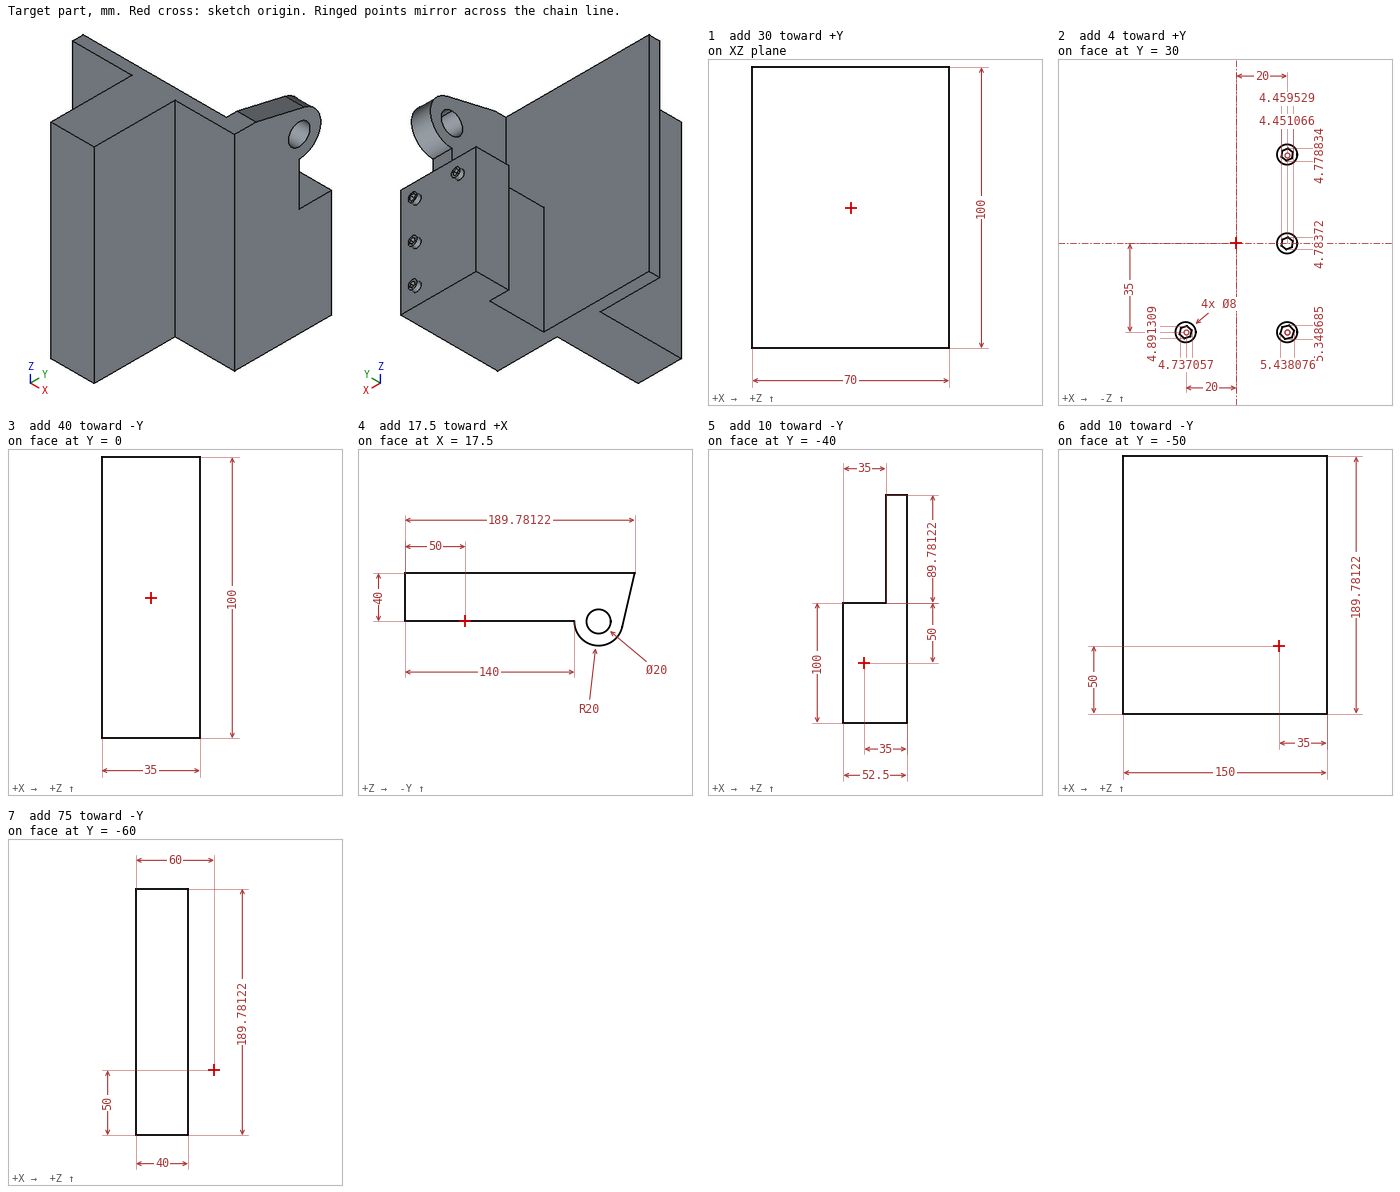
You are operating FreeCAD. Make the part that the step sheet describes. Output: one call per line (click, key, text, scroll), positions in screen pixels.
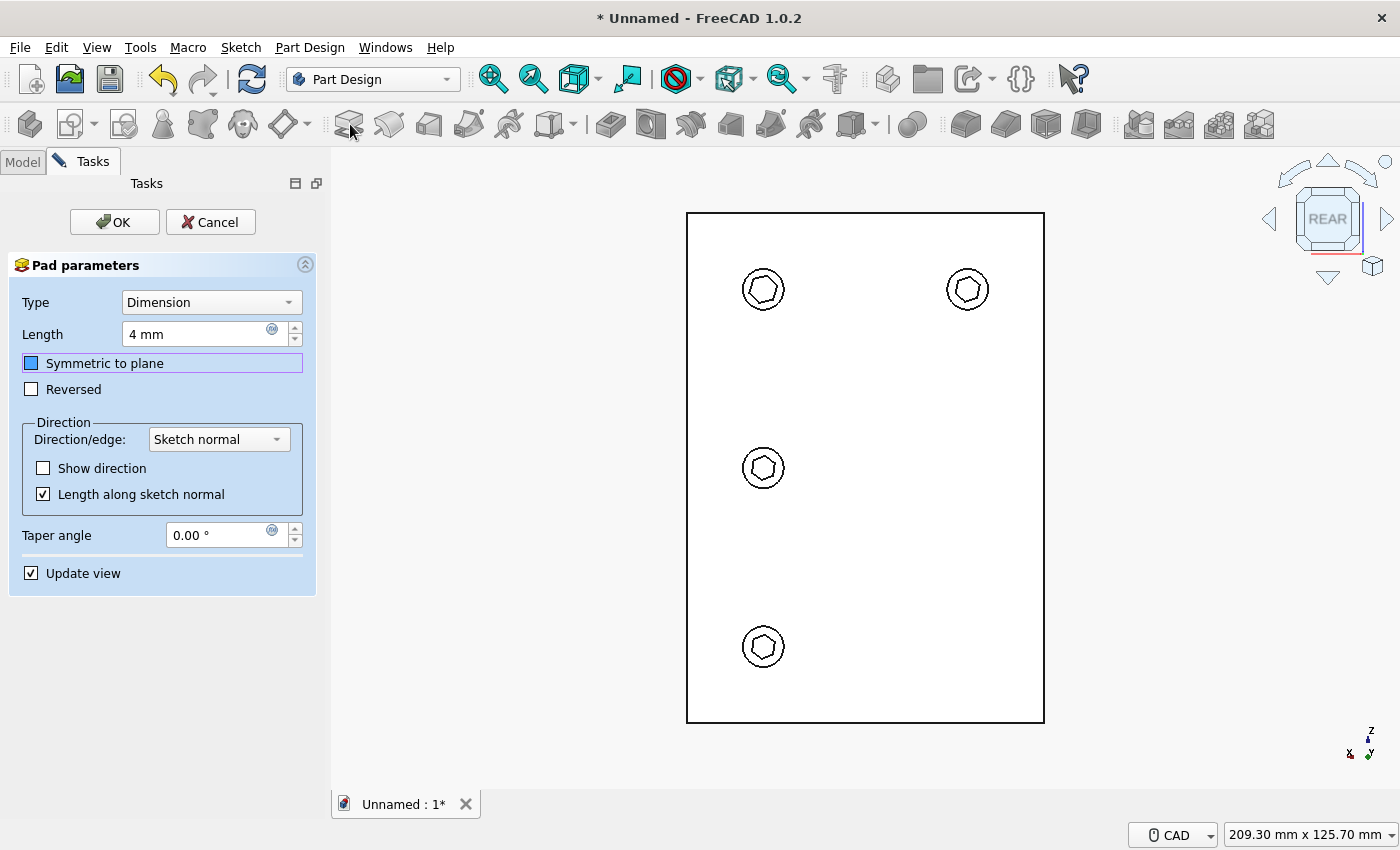
click(115, 222)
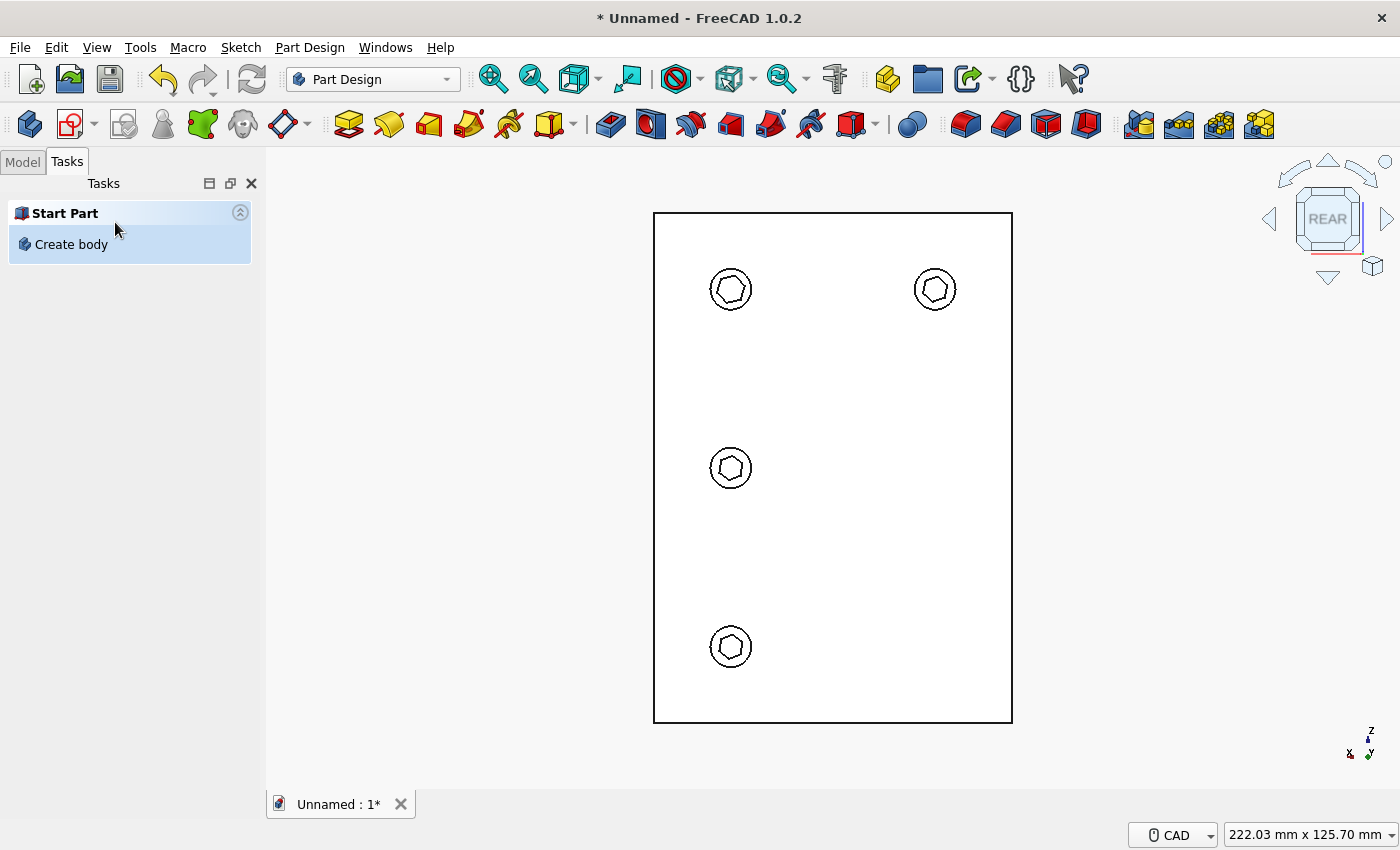
key(0)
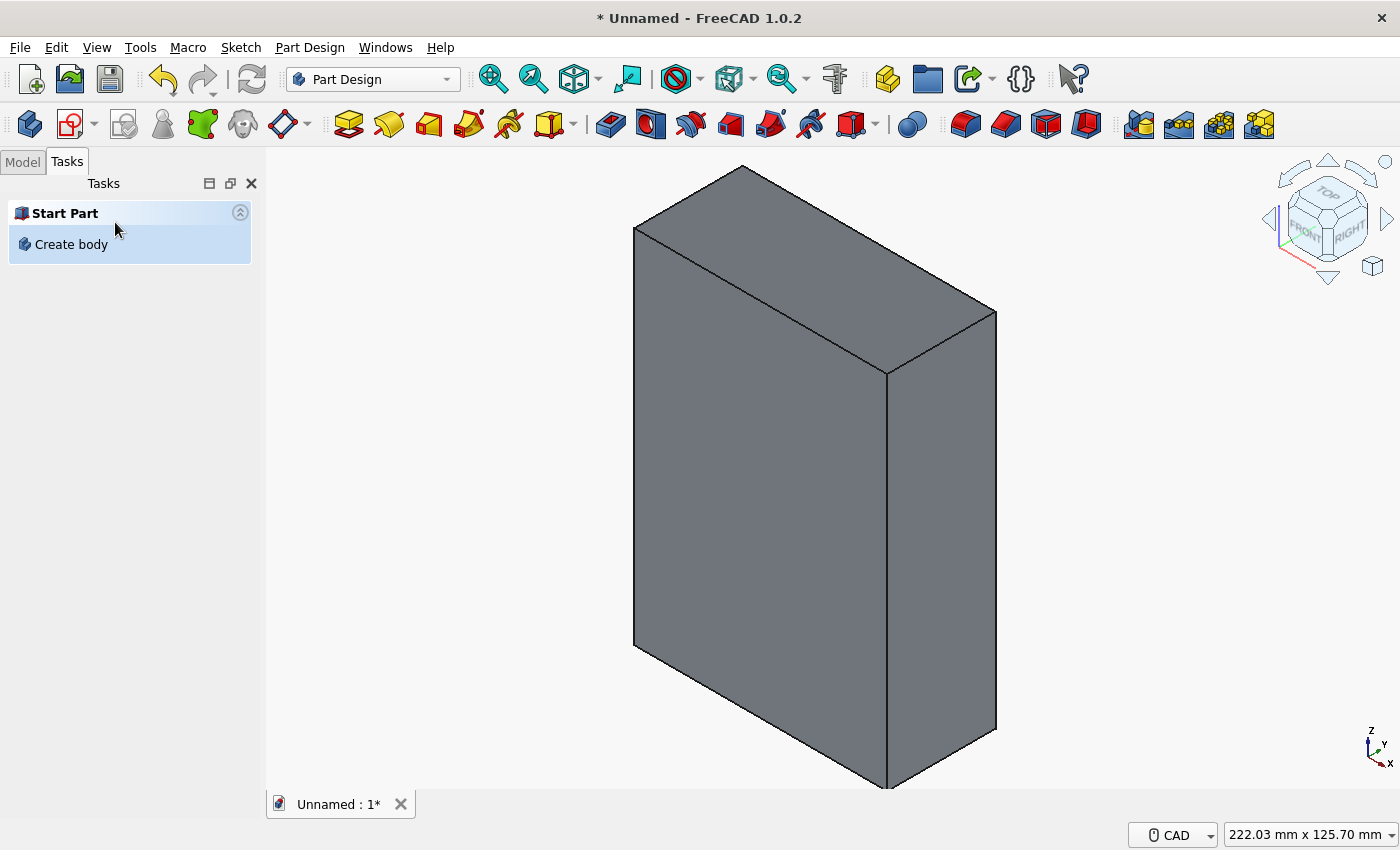
click(494, 80)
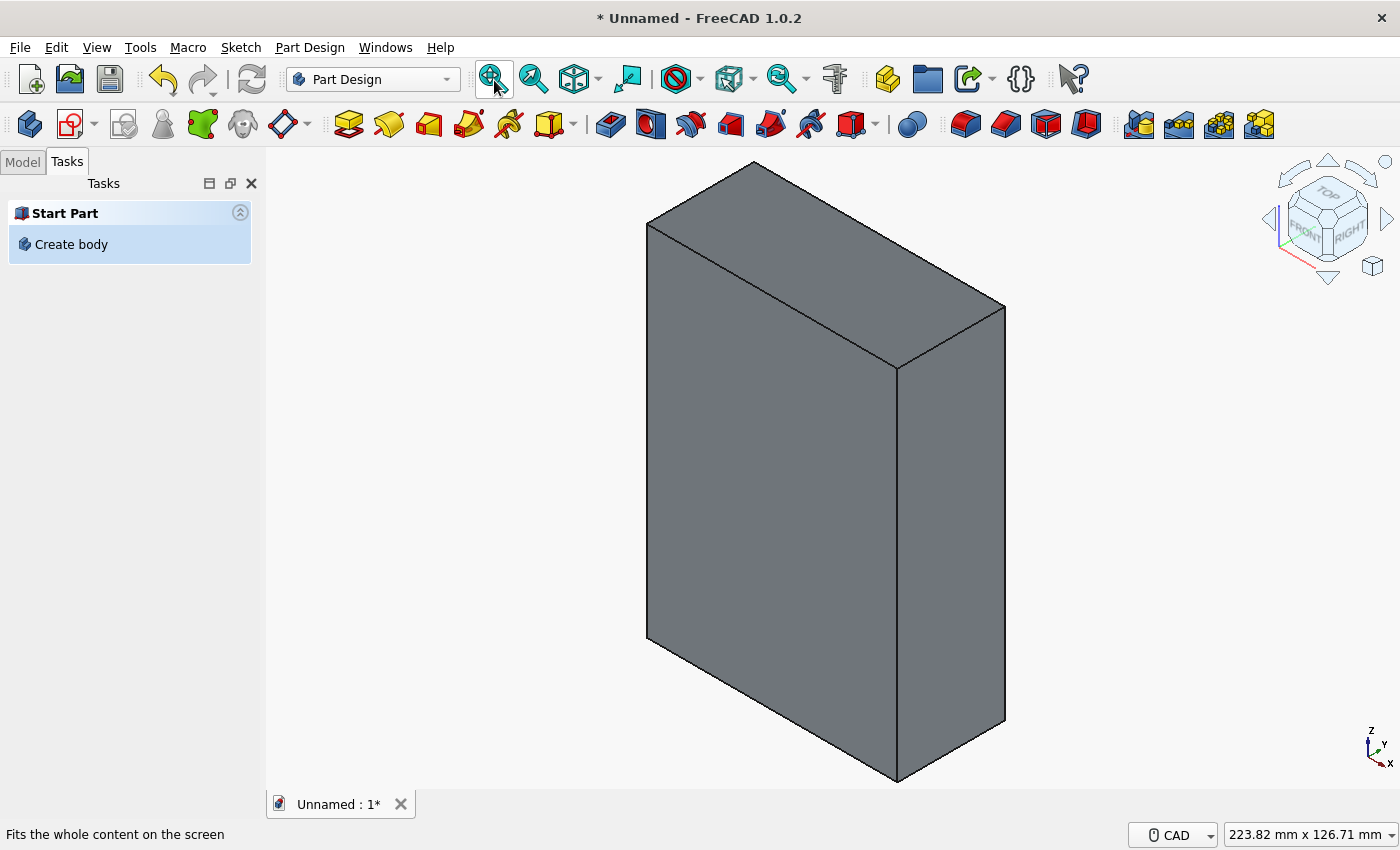
click(772, 443)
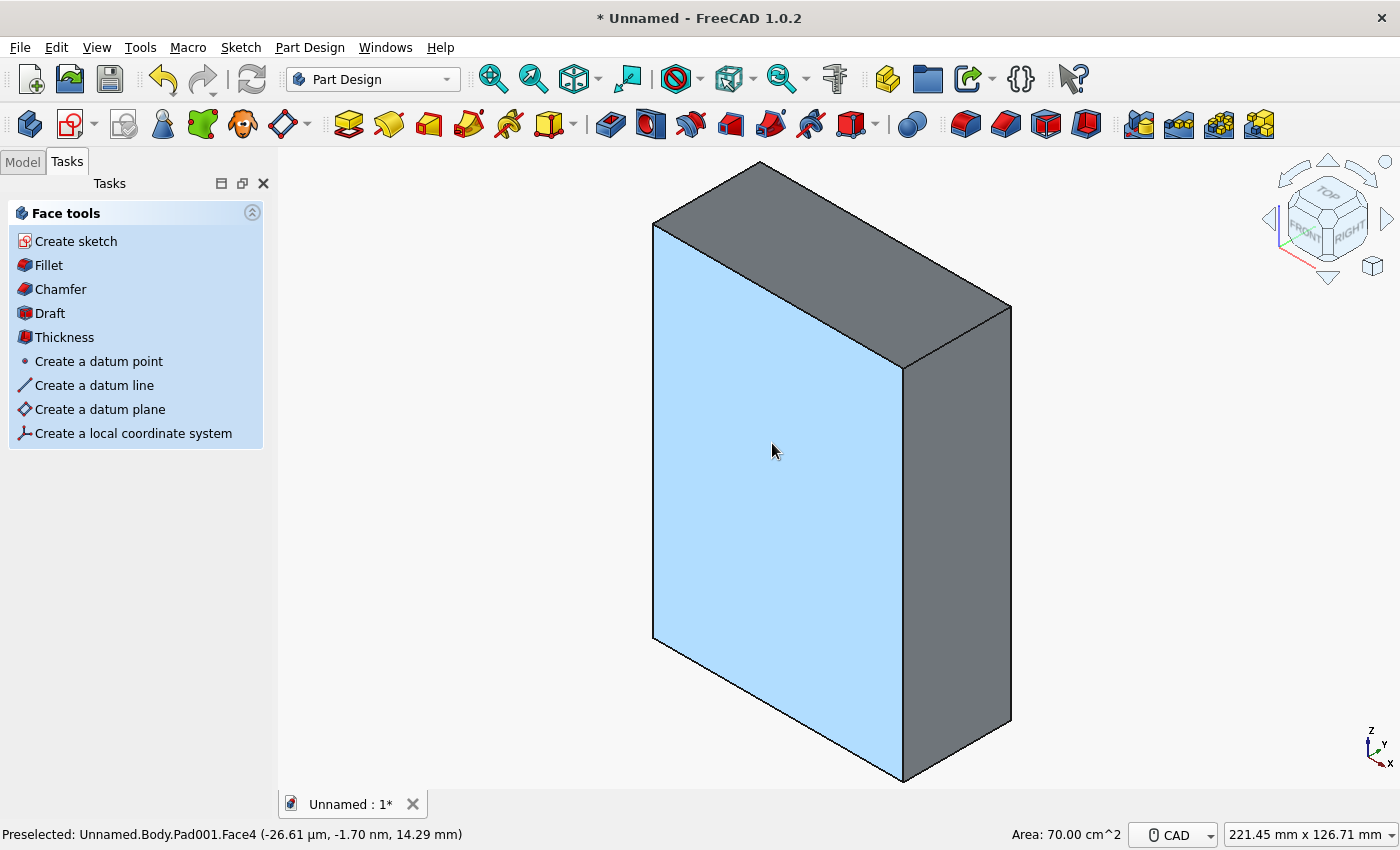
click(70, 124)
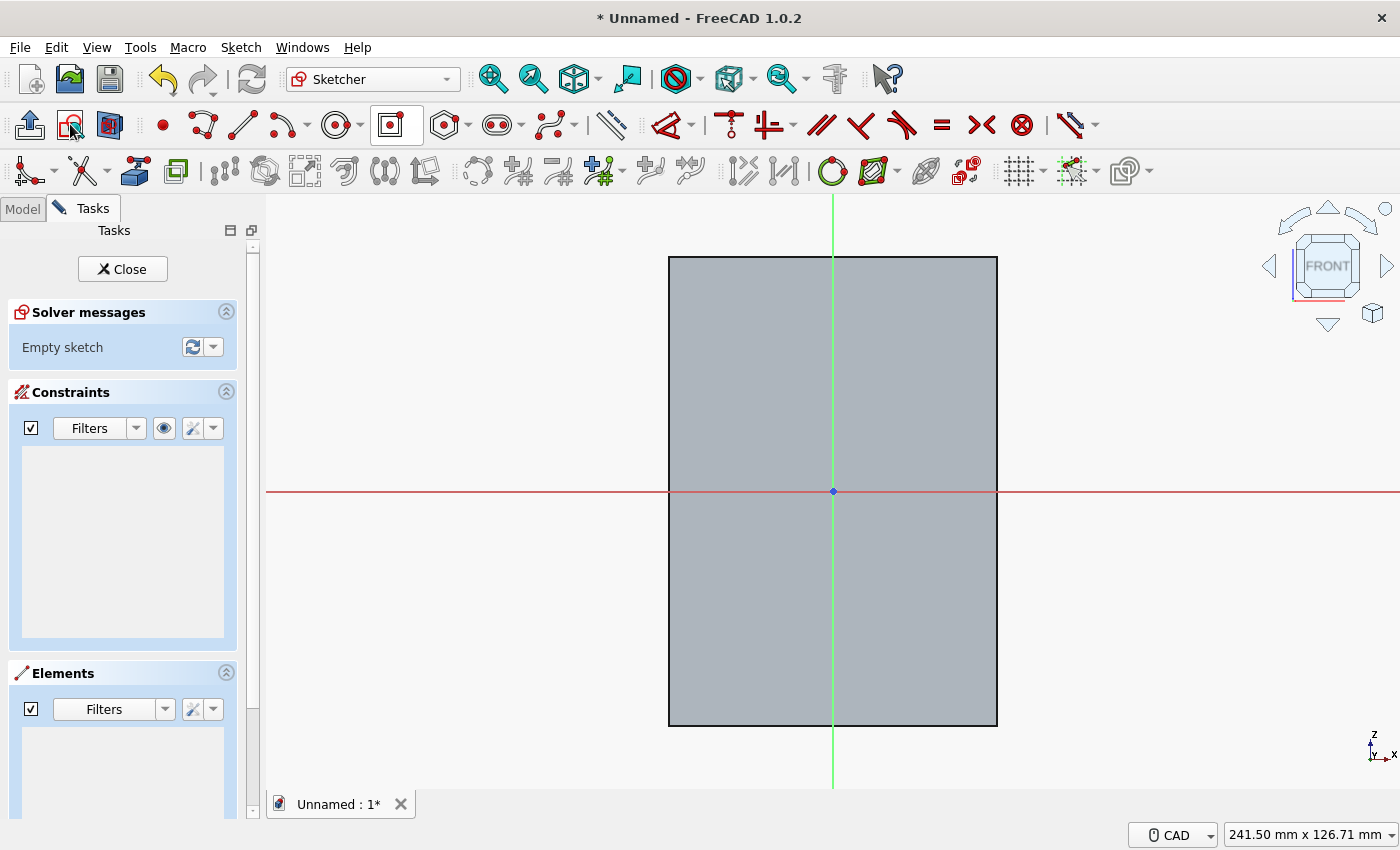
click(390, 126)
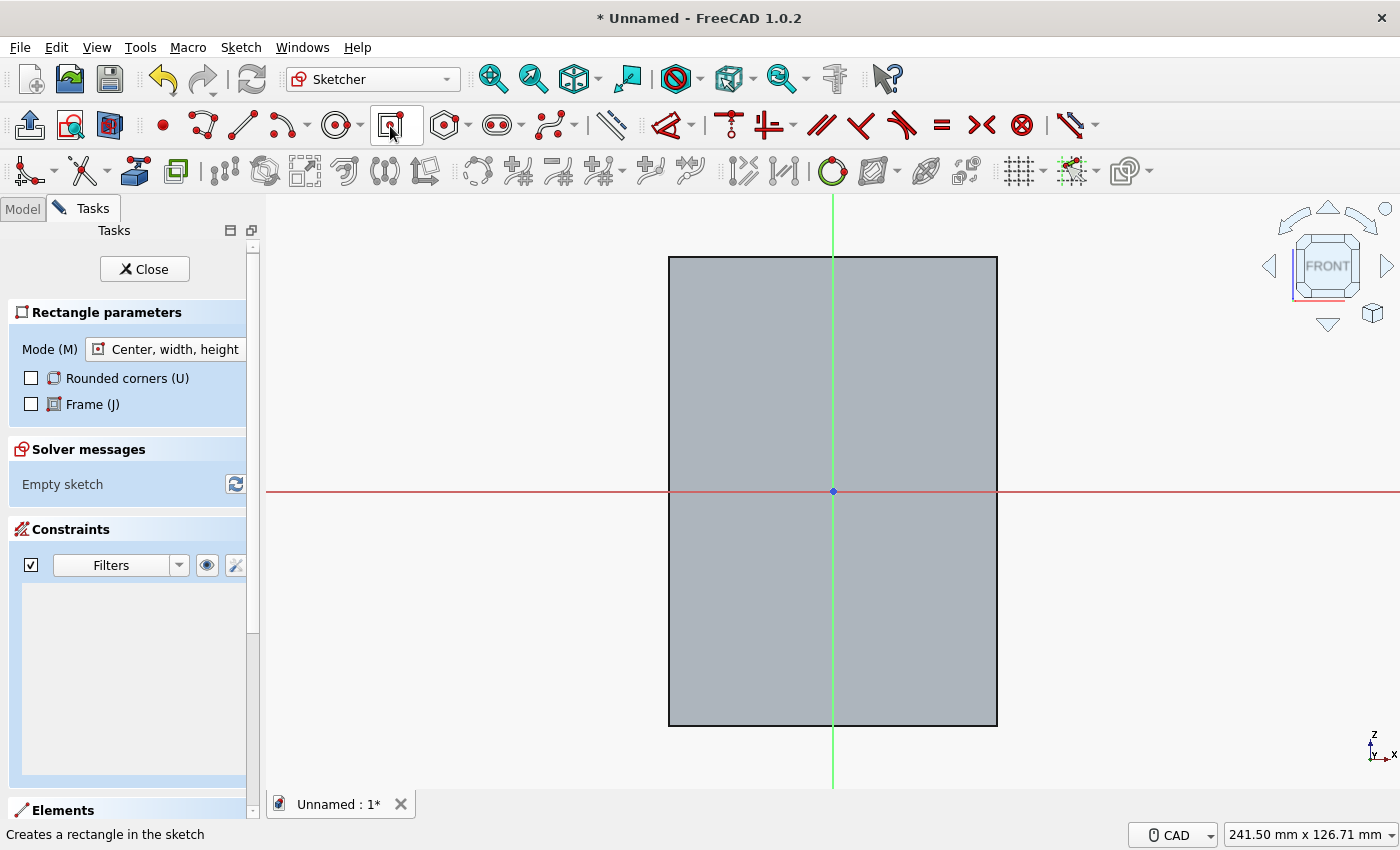
click(833, 492)
move(915, 257)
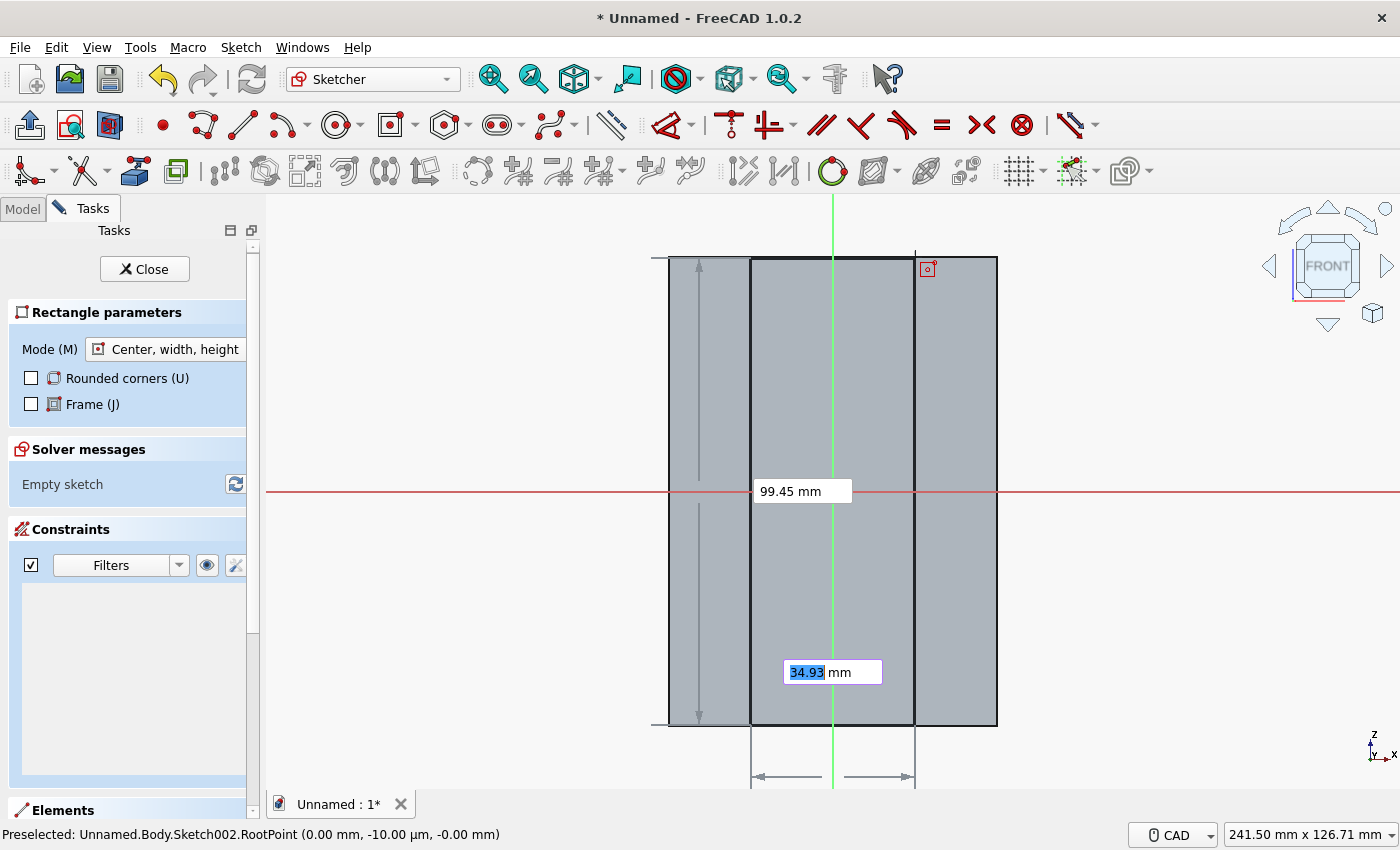
text(35)
key(Tab)
text(100)
key(Return)
key(Escape)